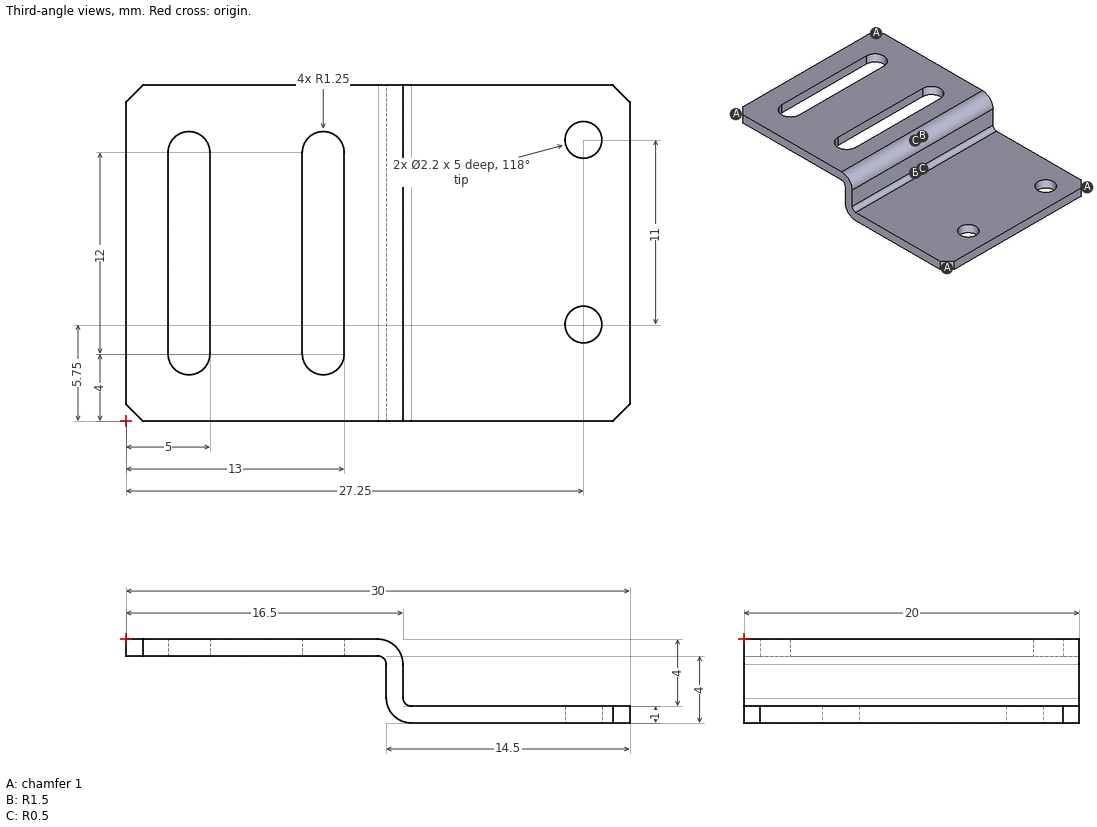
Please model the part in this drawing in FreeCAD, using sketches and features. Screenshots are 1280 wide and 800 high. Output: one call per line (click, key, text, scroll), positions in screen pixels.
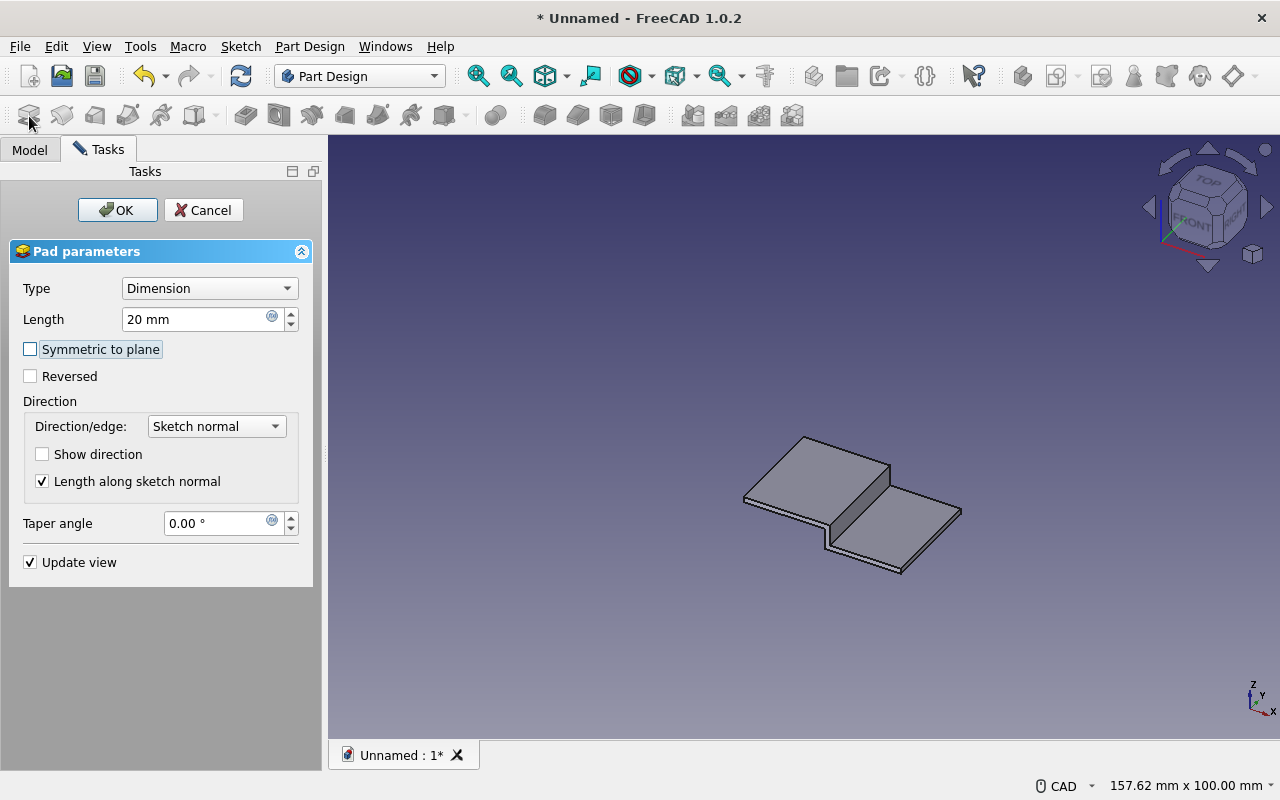
click(31, 376)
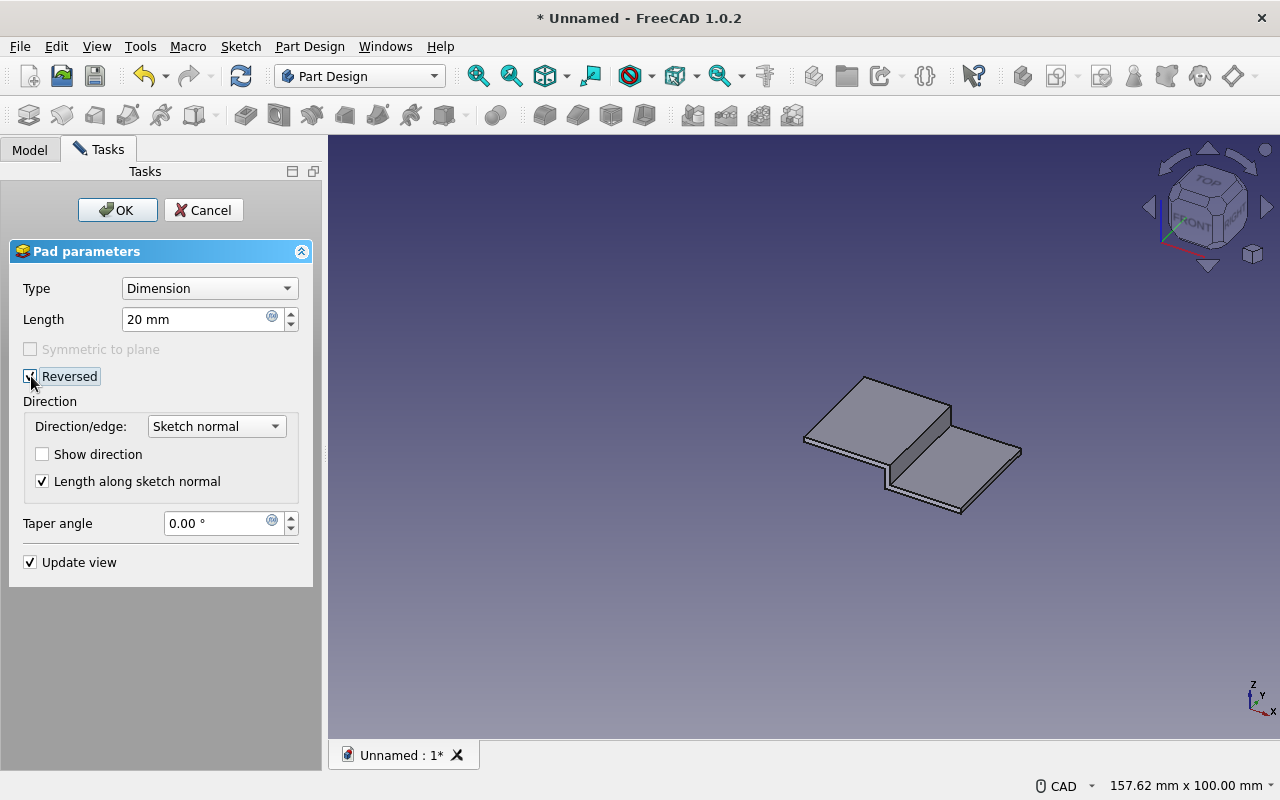
click(118, 210)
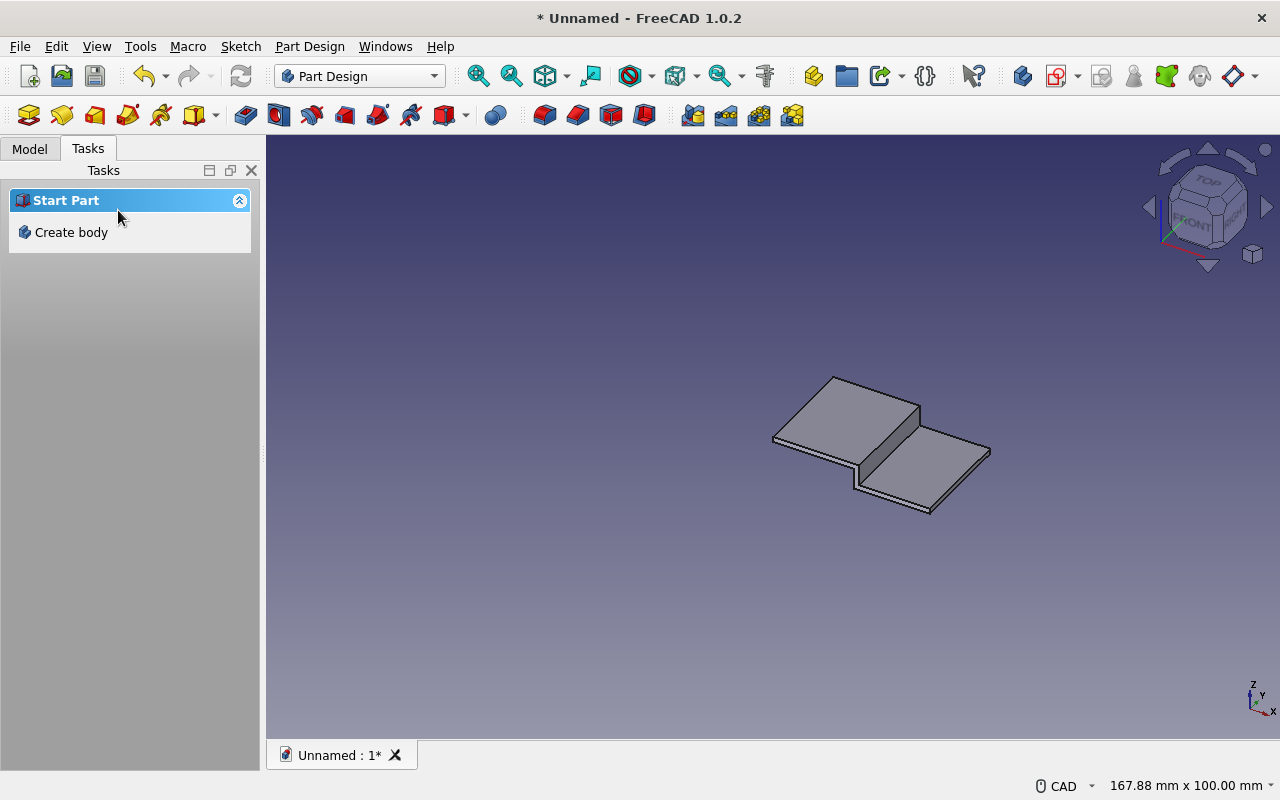
click(479, 76)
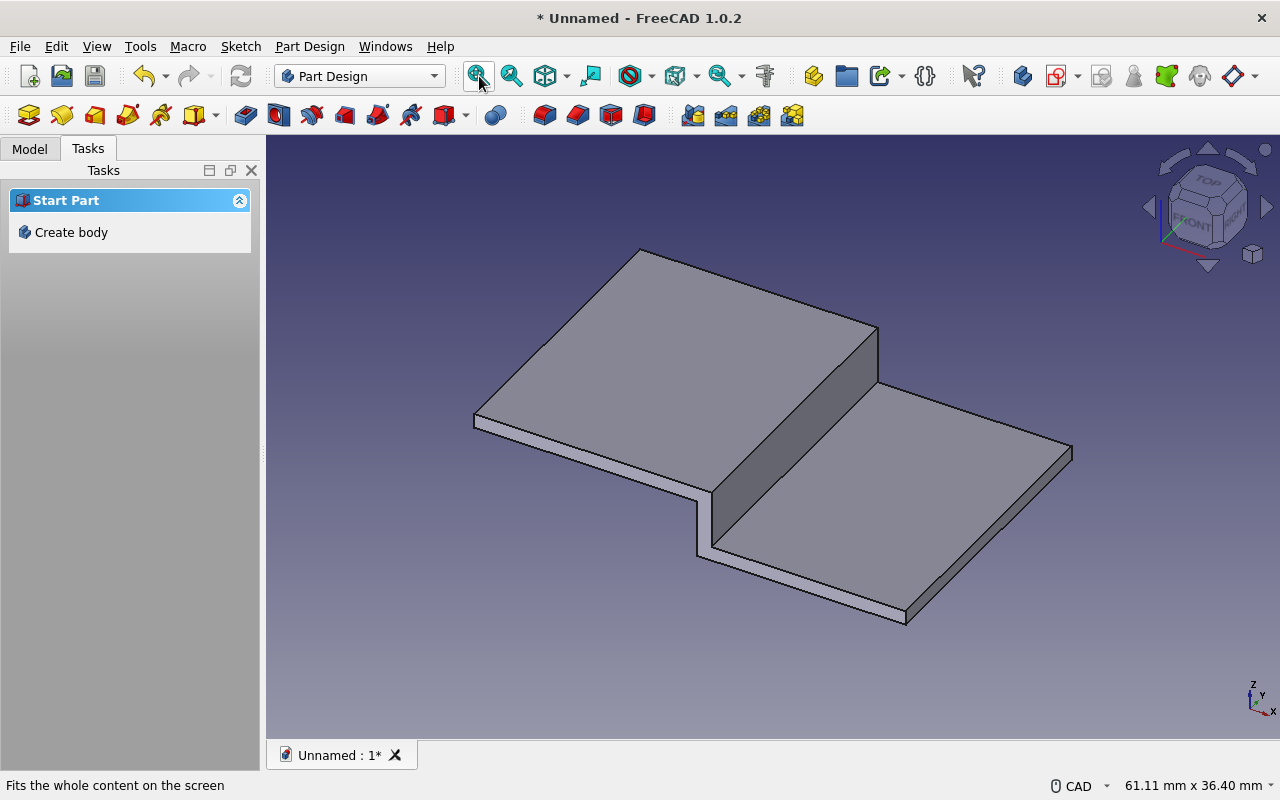
key(5)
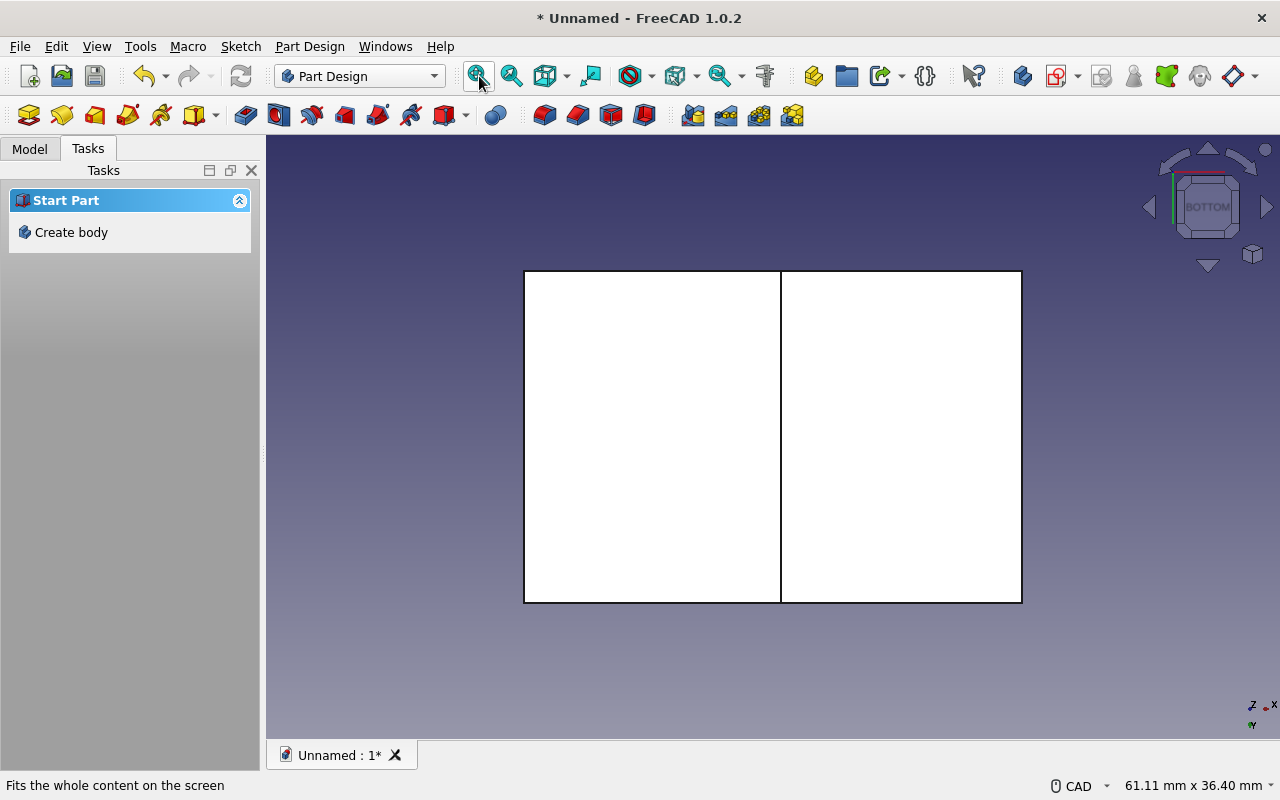
click(902, 436)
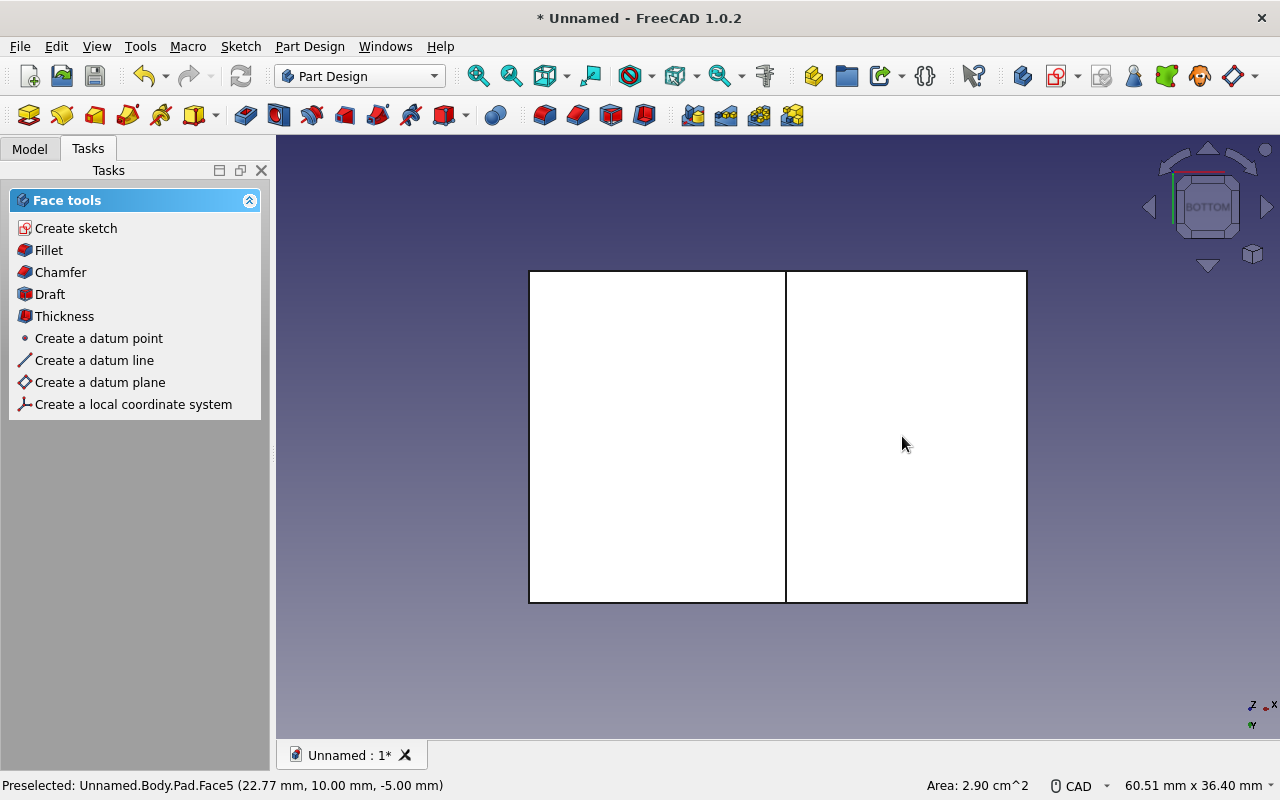
click(1056, 76)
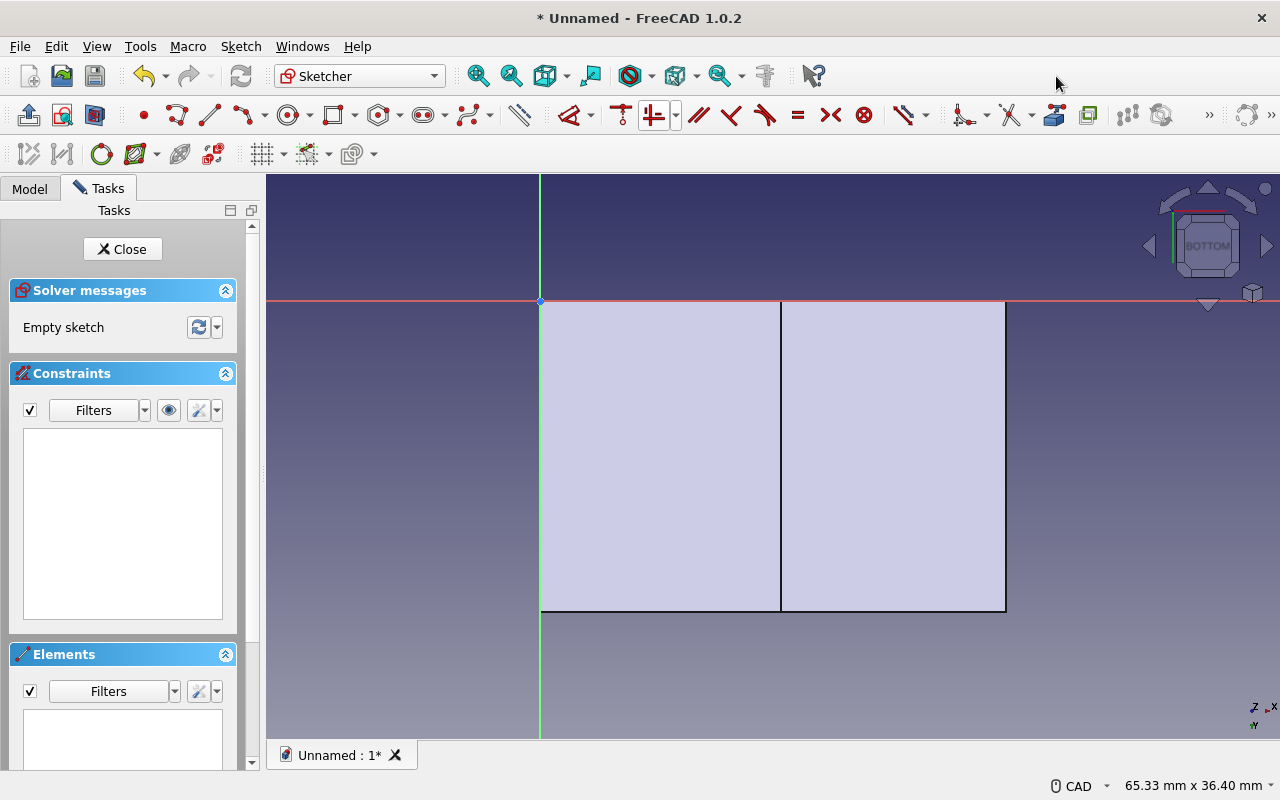
click(422, 116)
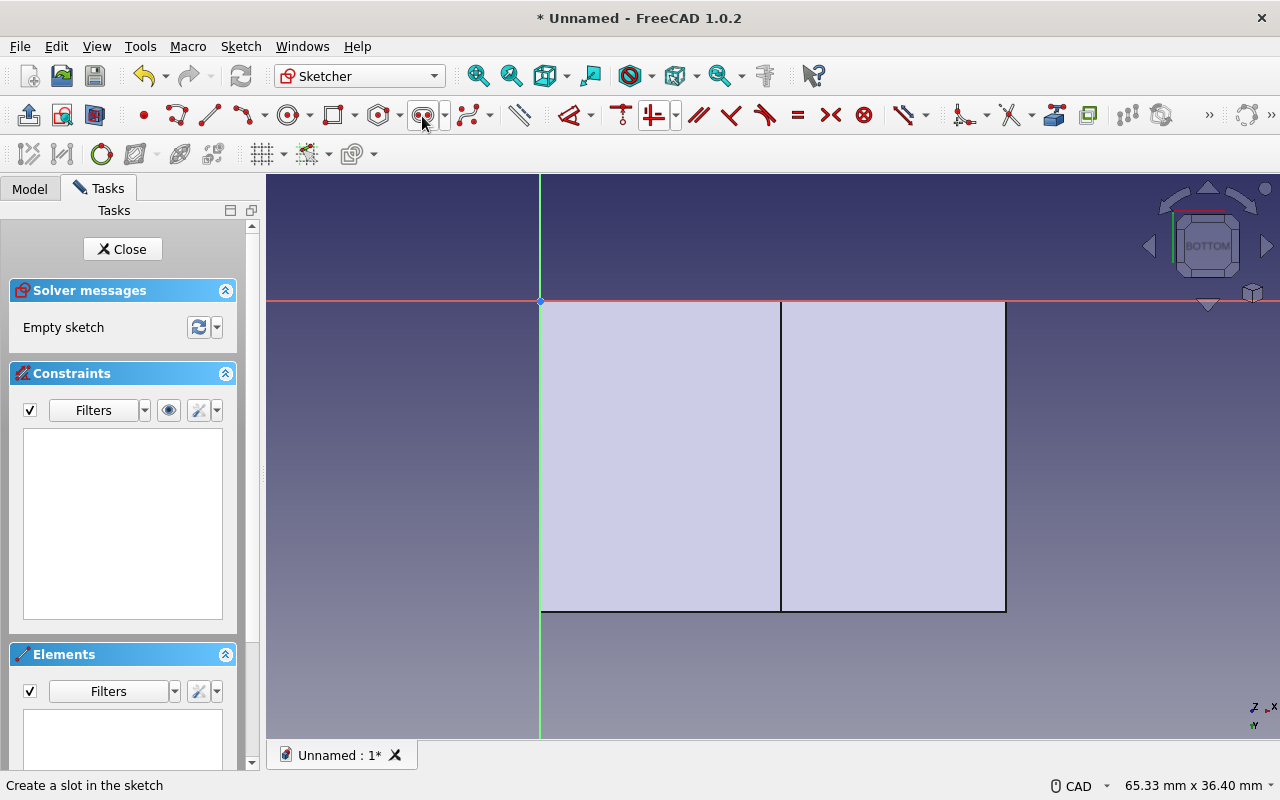
click(723, 550)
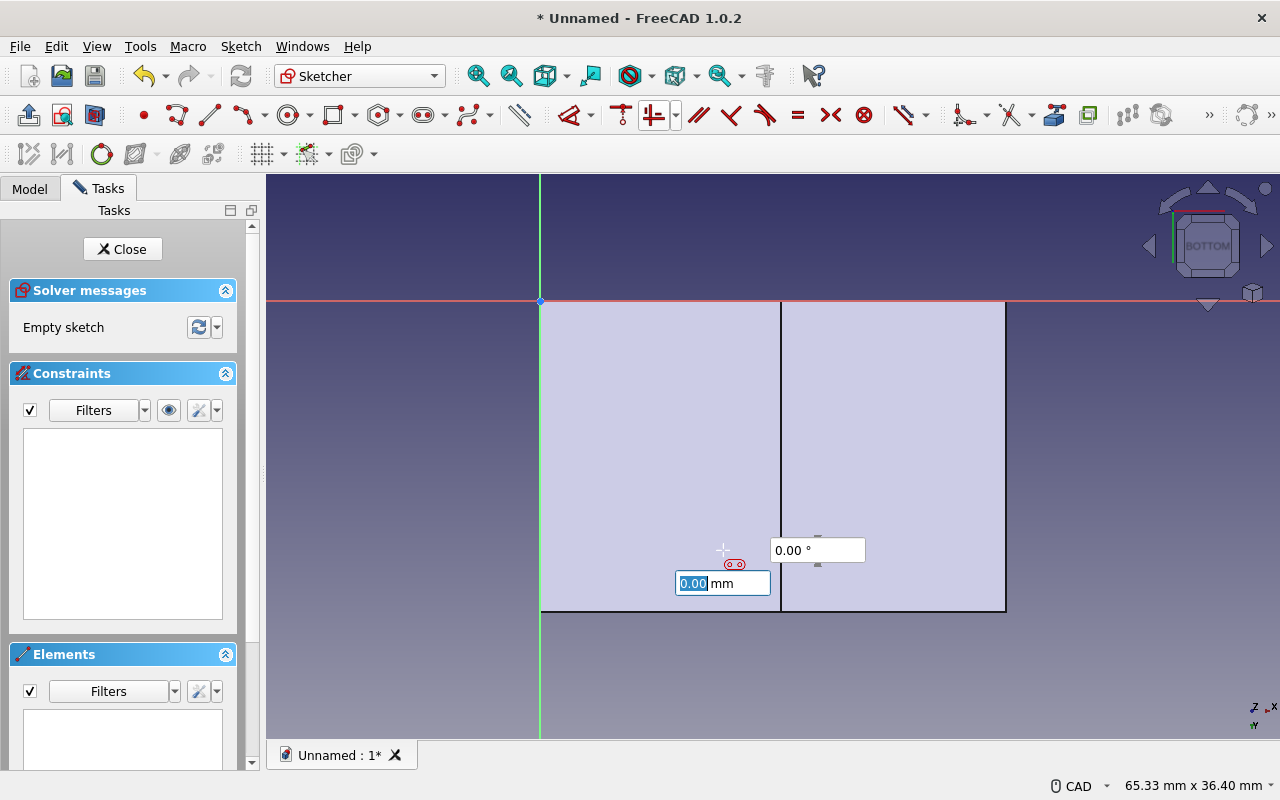
click(723, 363)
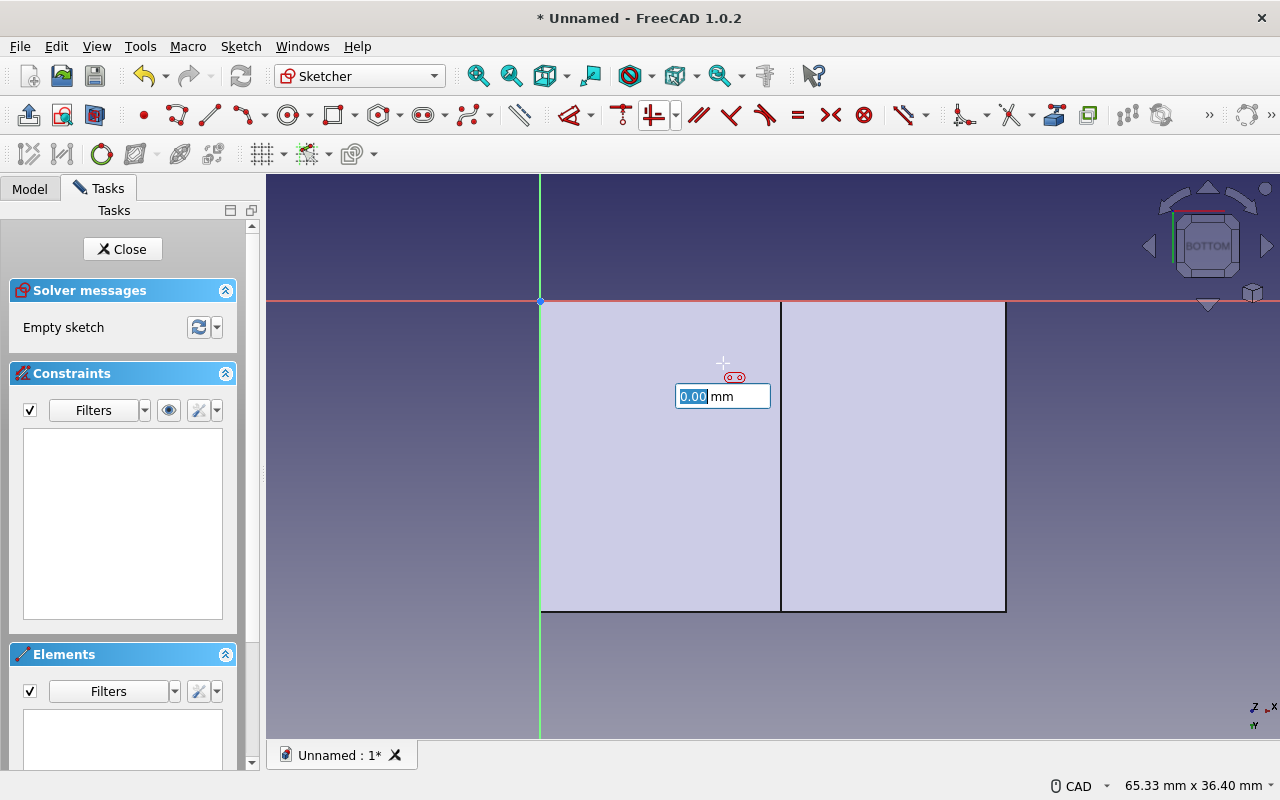
click(703, 456)